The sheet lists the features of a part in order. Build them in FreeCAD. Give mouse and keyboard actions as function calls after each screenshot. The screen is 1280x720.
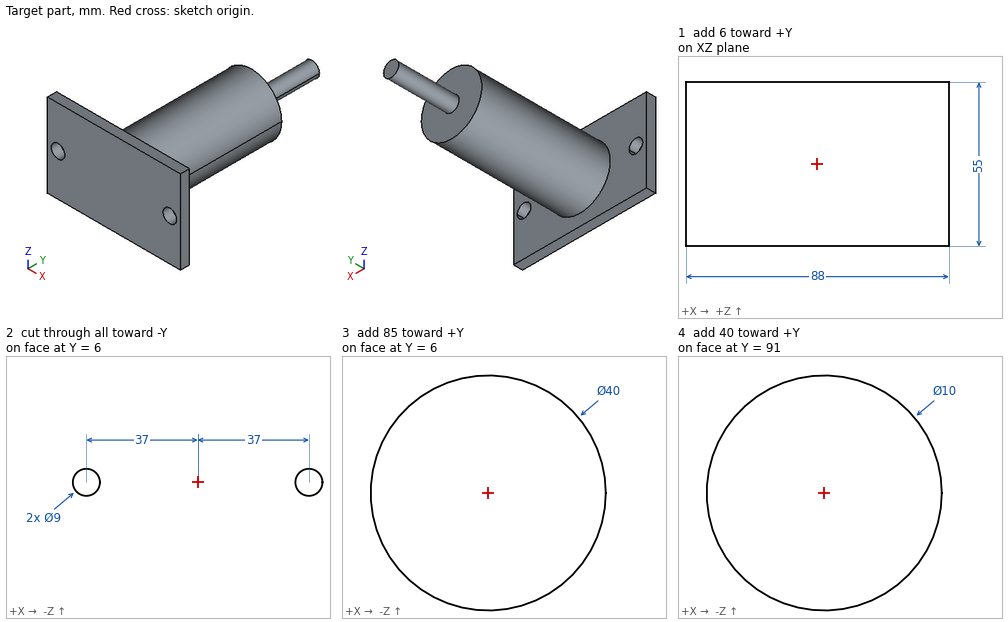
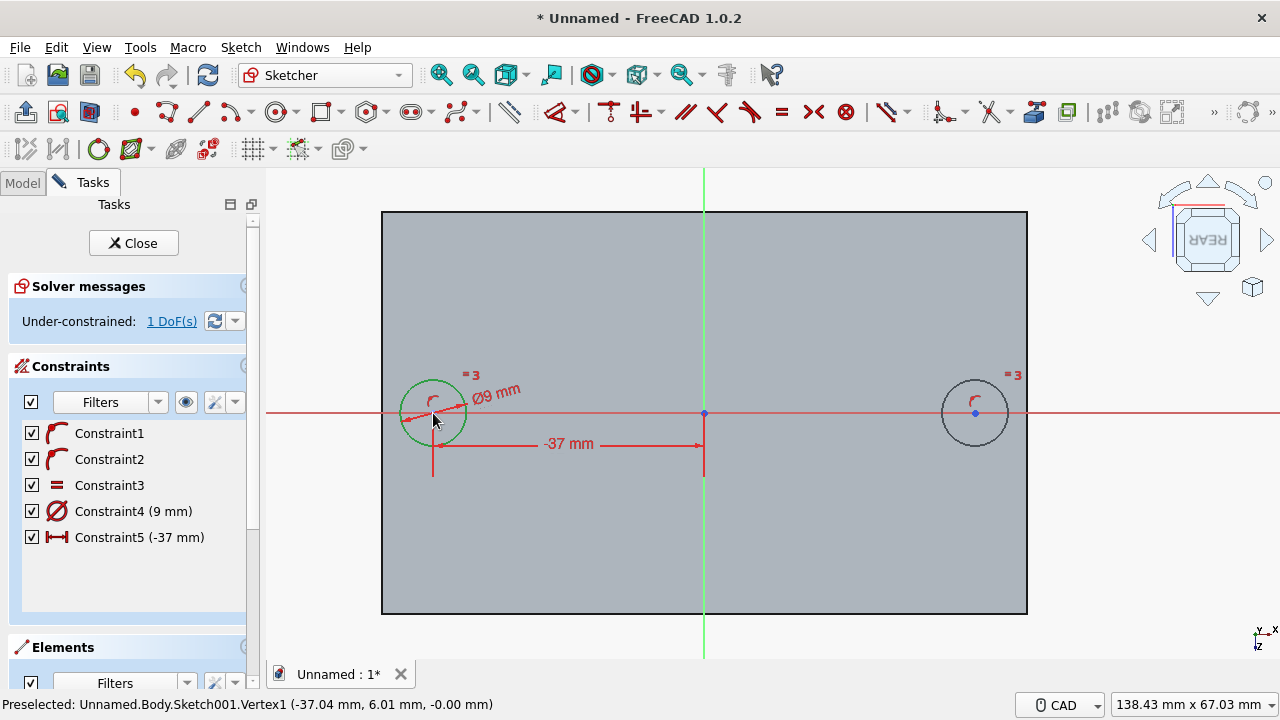
click(975, 413)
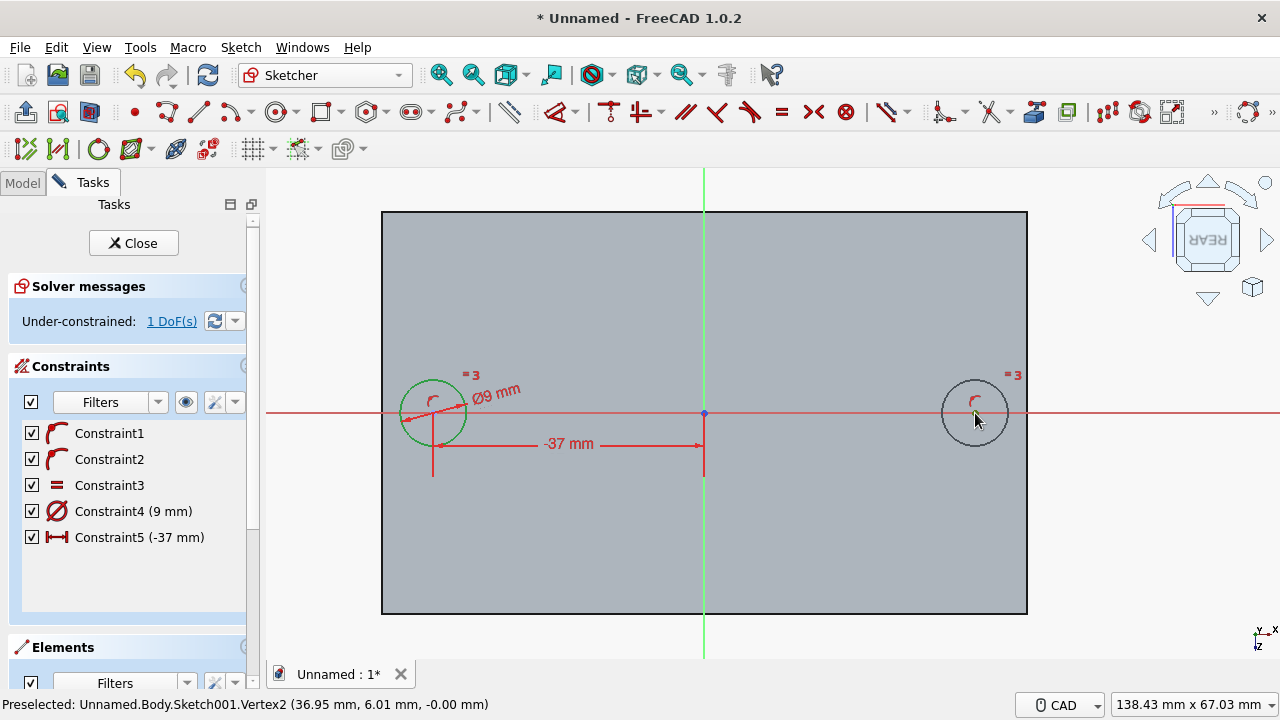
key(l)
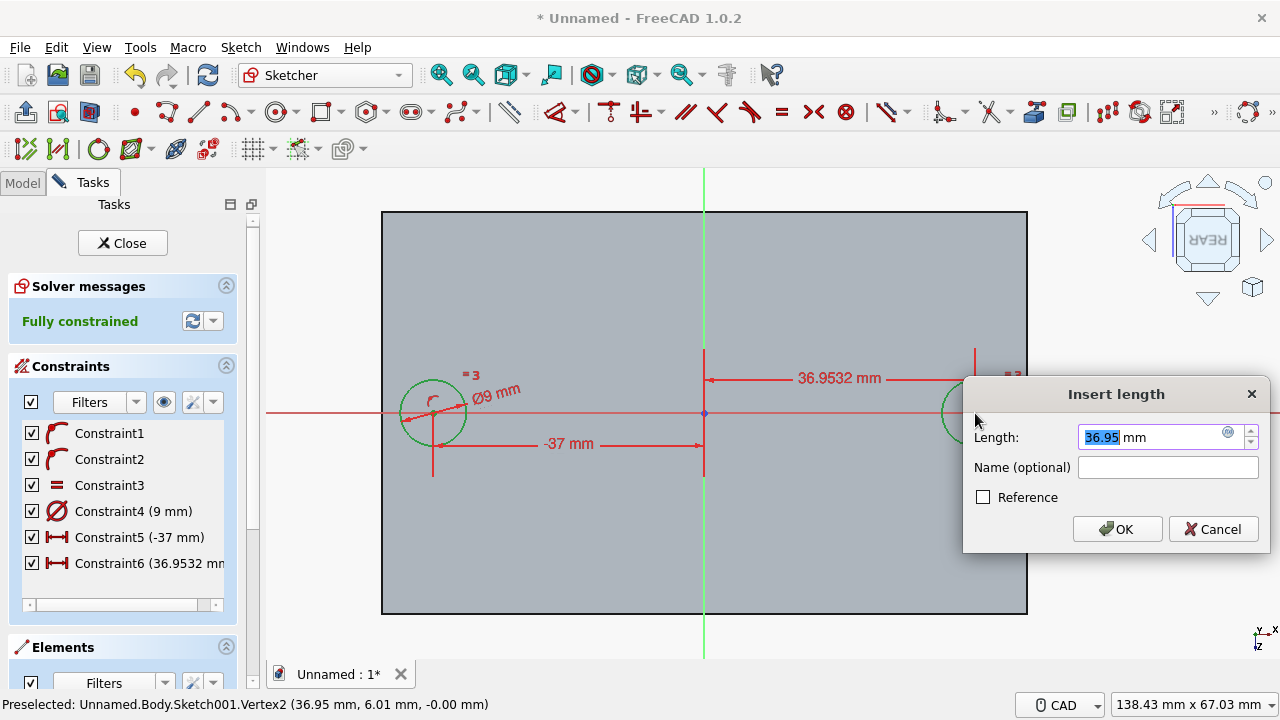
text(37)
key(Return)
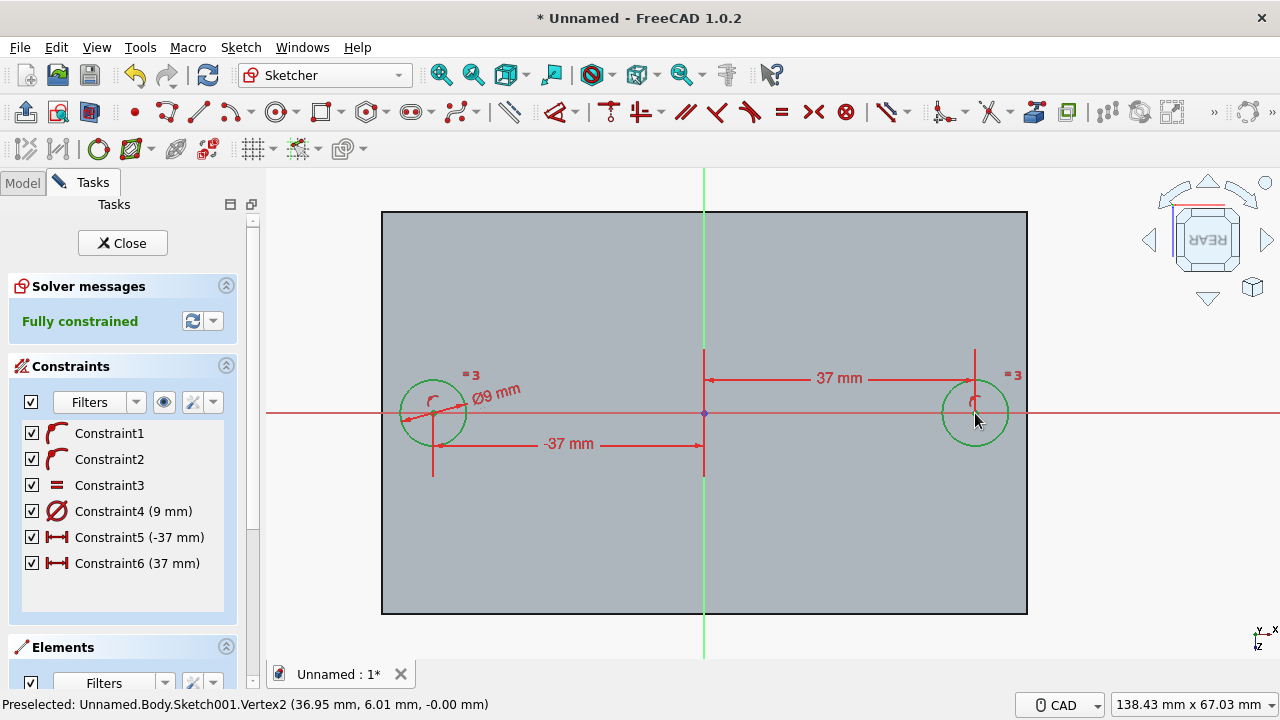
click(123, 243)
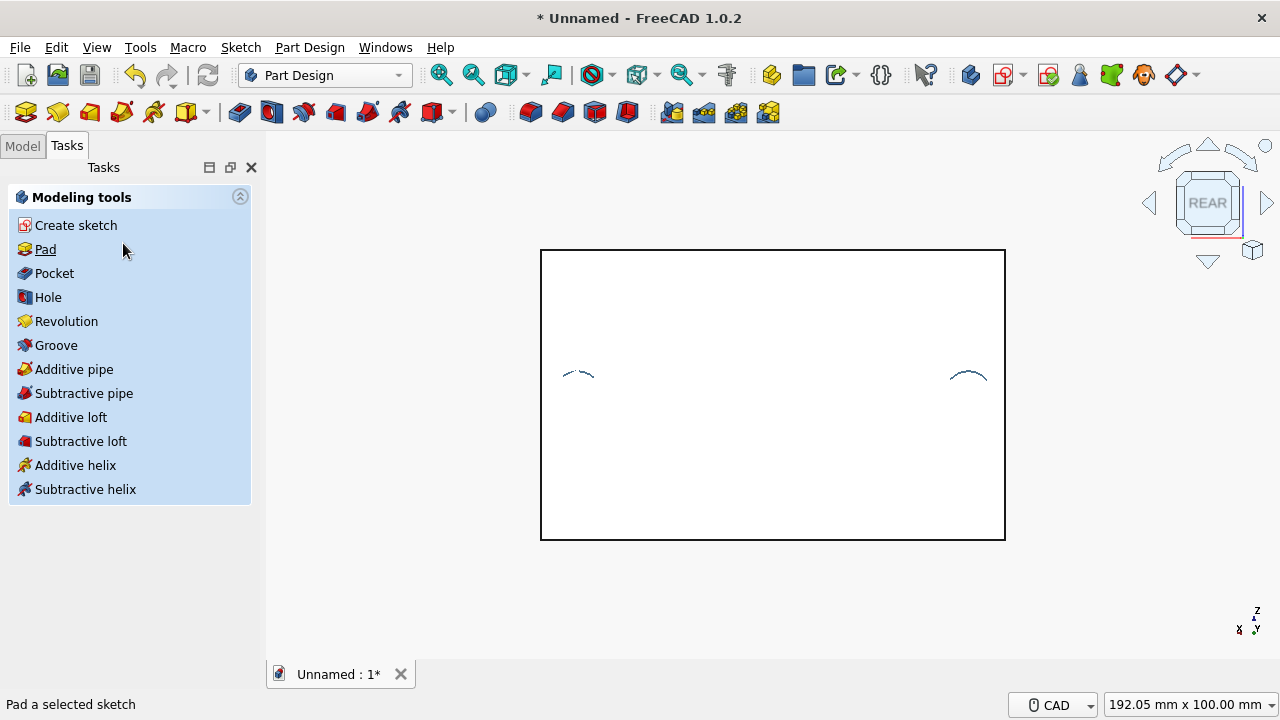
click(240, 112)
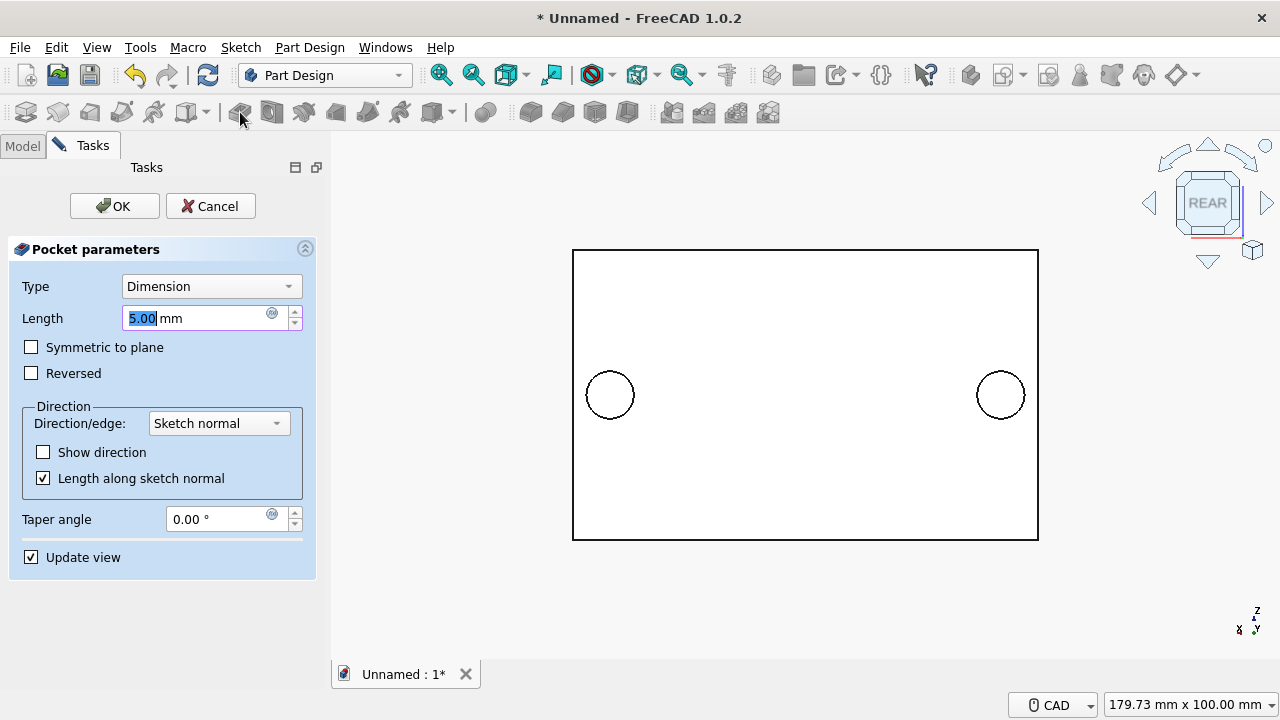
click(212, 286)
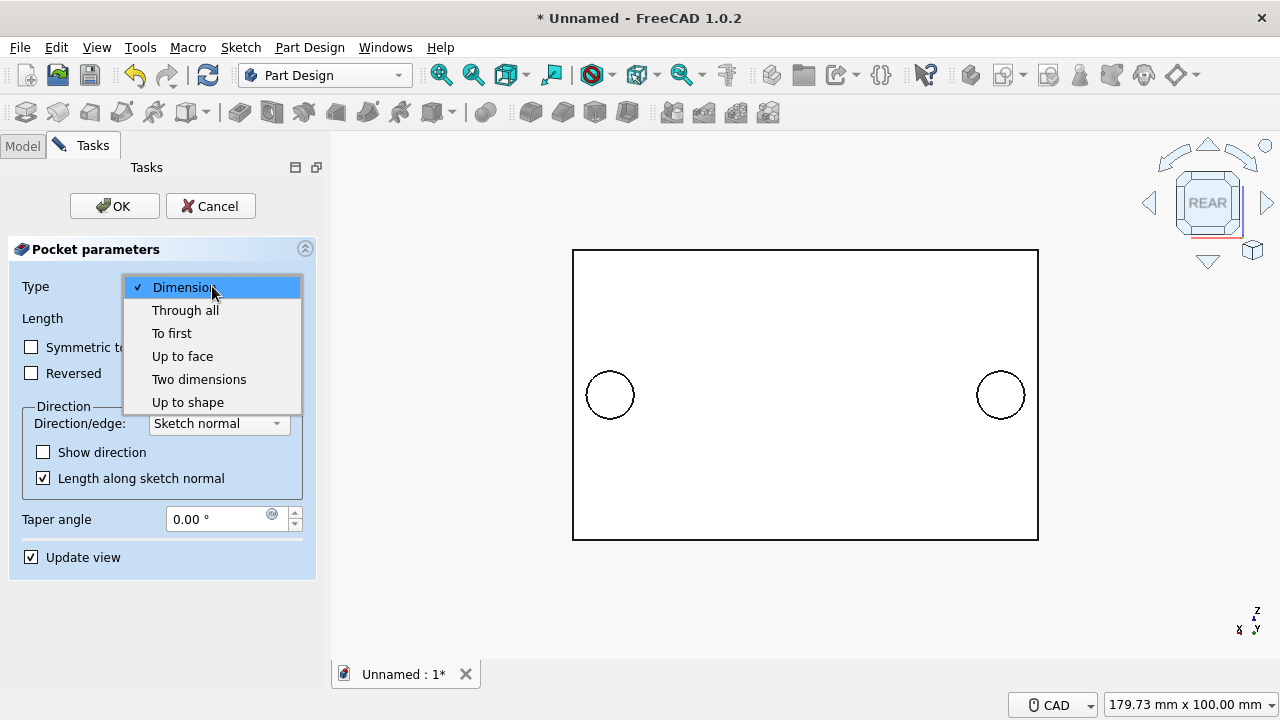
click(212, 310)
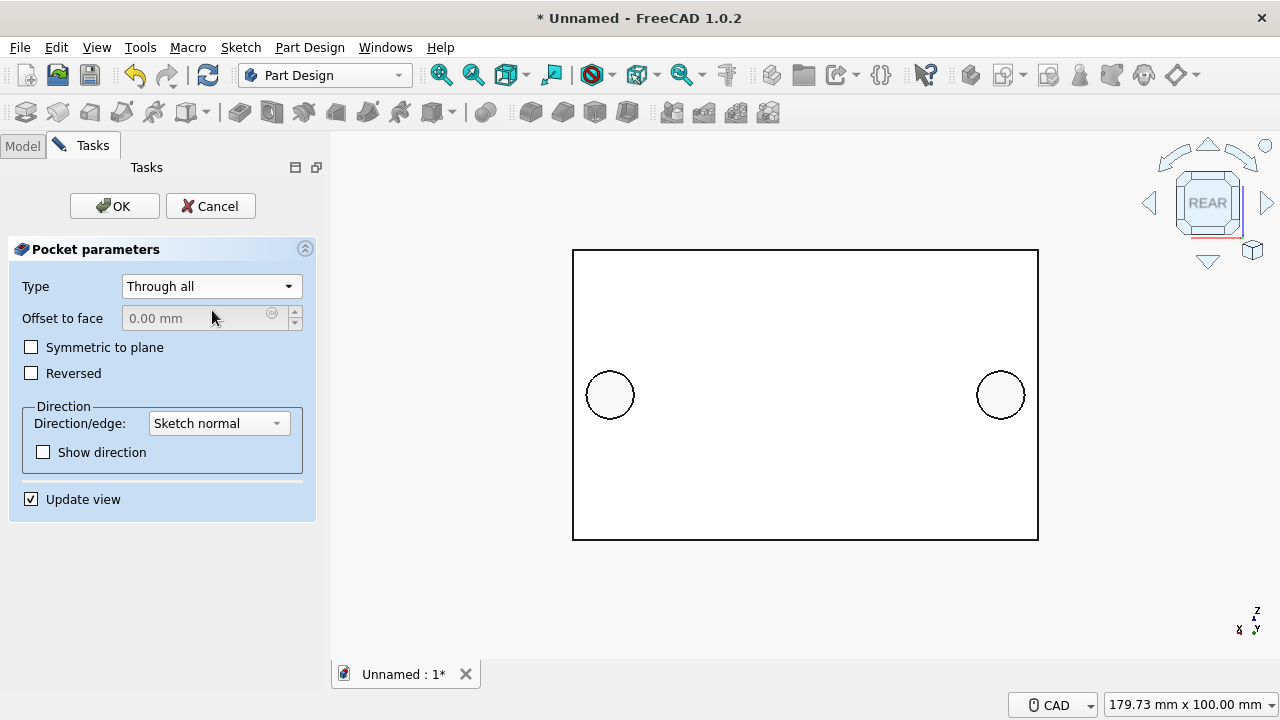
click(115, 206)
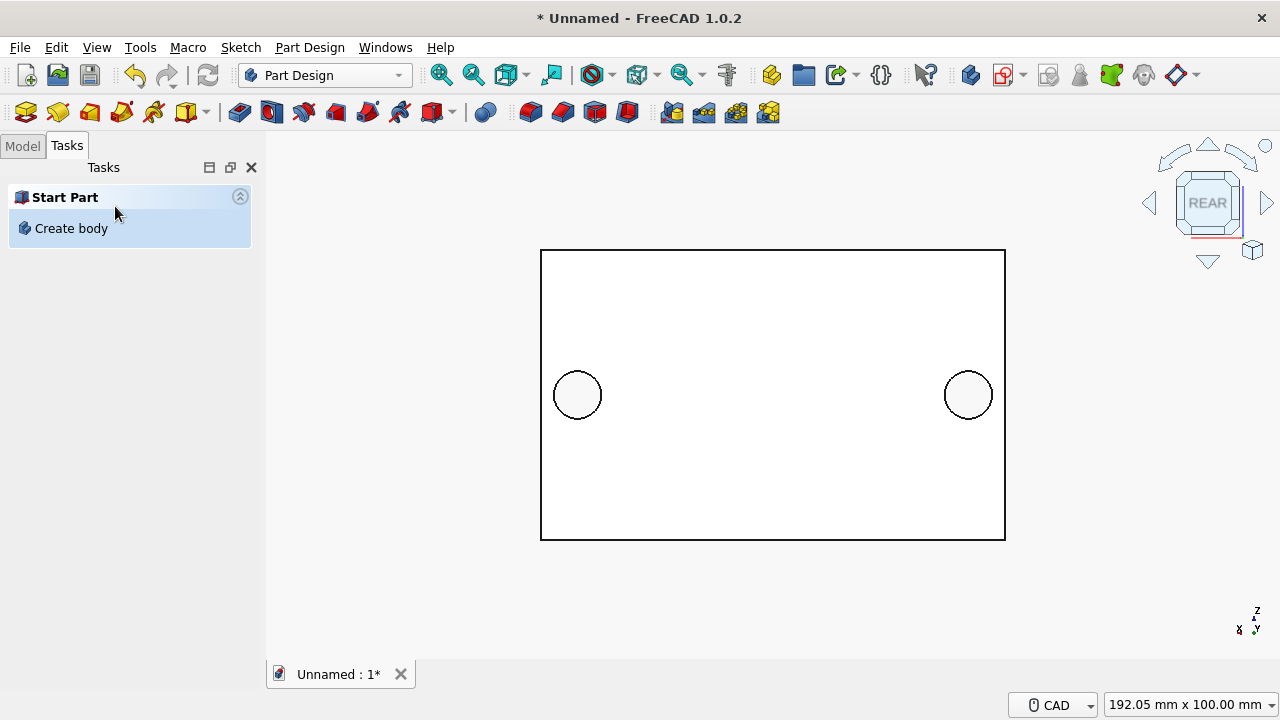
click(773, 394)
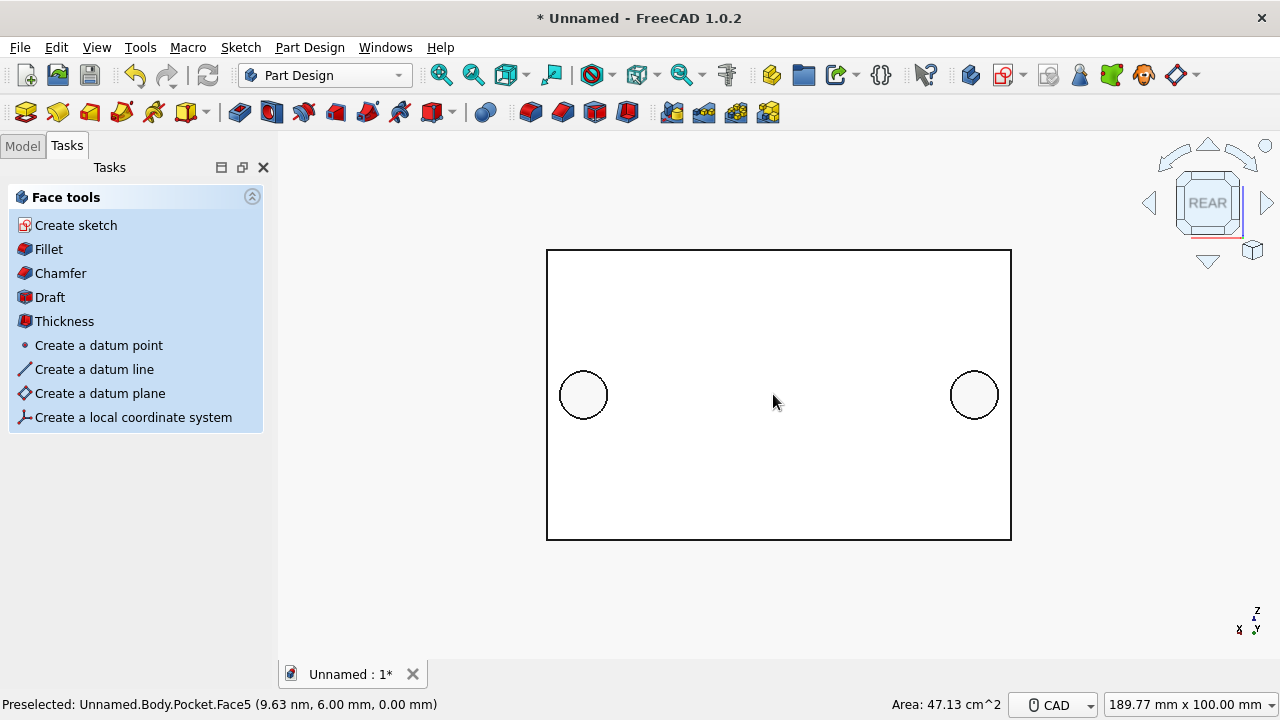
click(1004, 76)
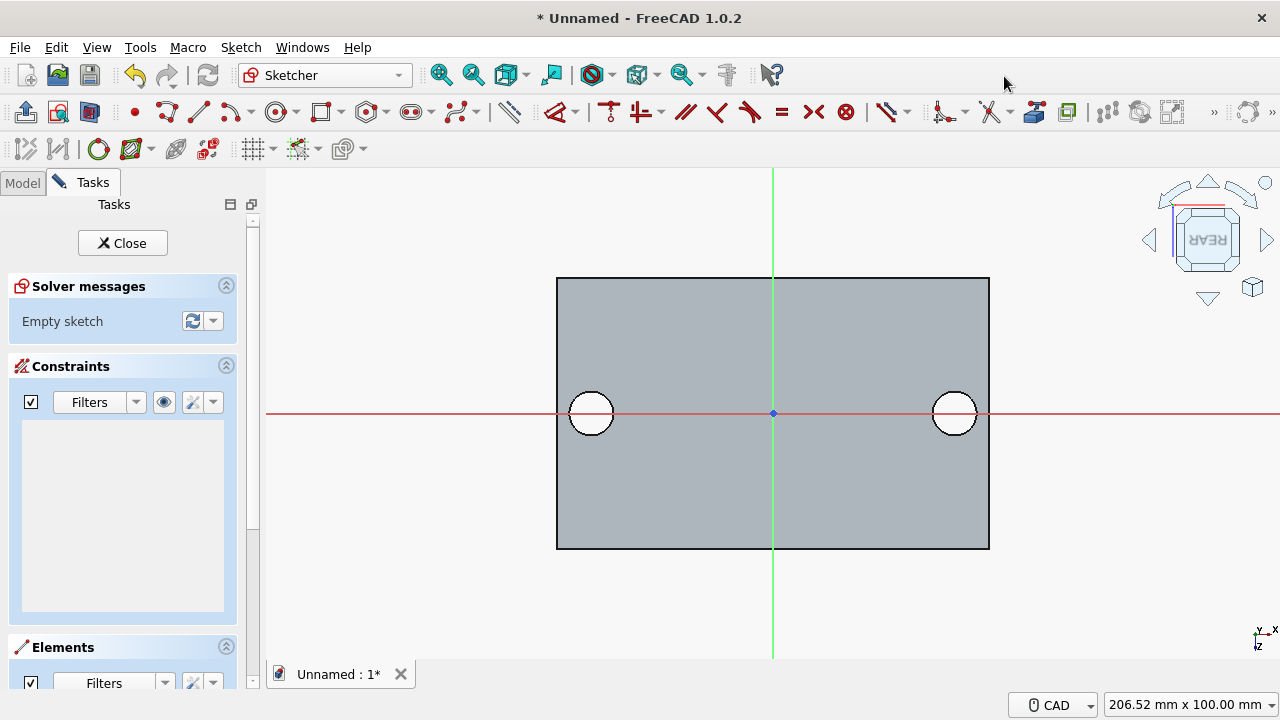
scroll(912, 413, up, 2)